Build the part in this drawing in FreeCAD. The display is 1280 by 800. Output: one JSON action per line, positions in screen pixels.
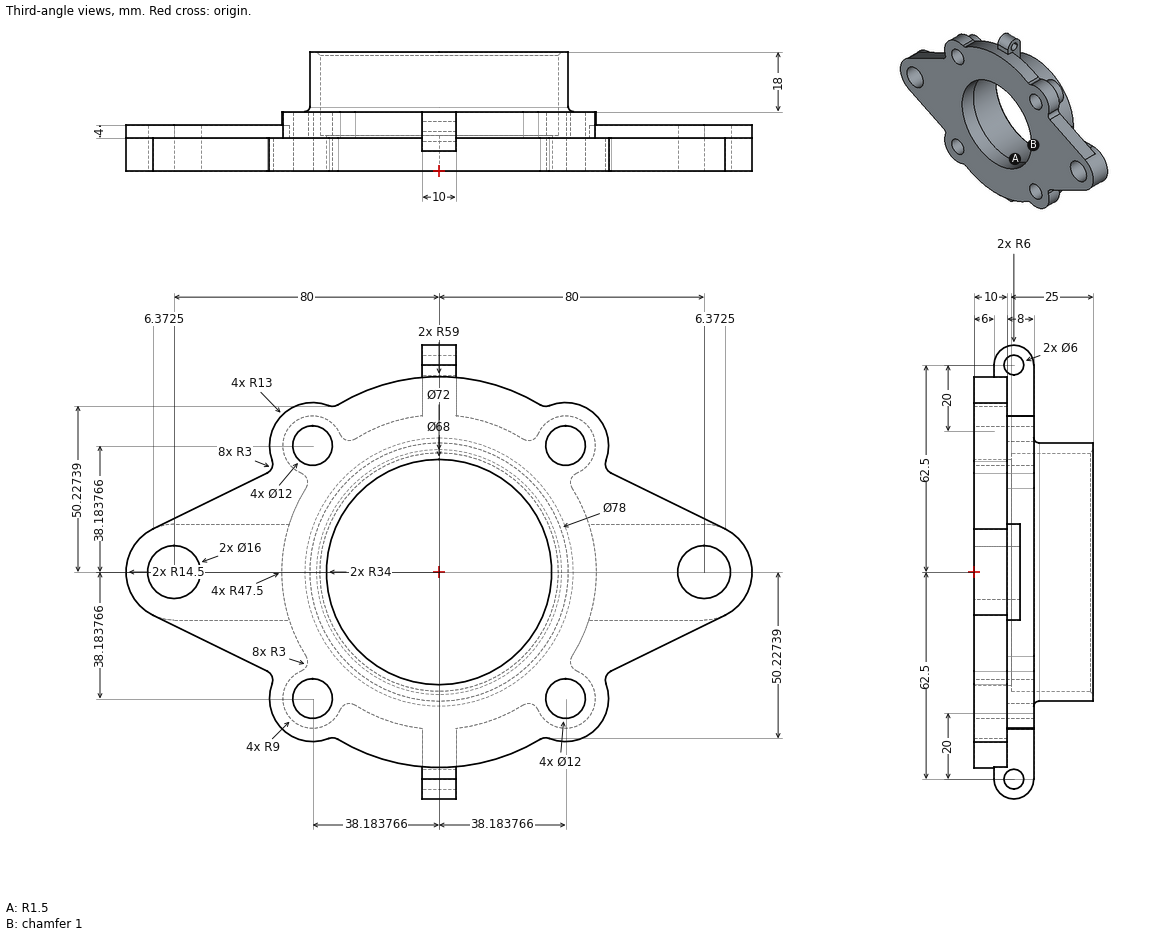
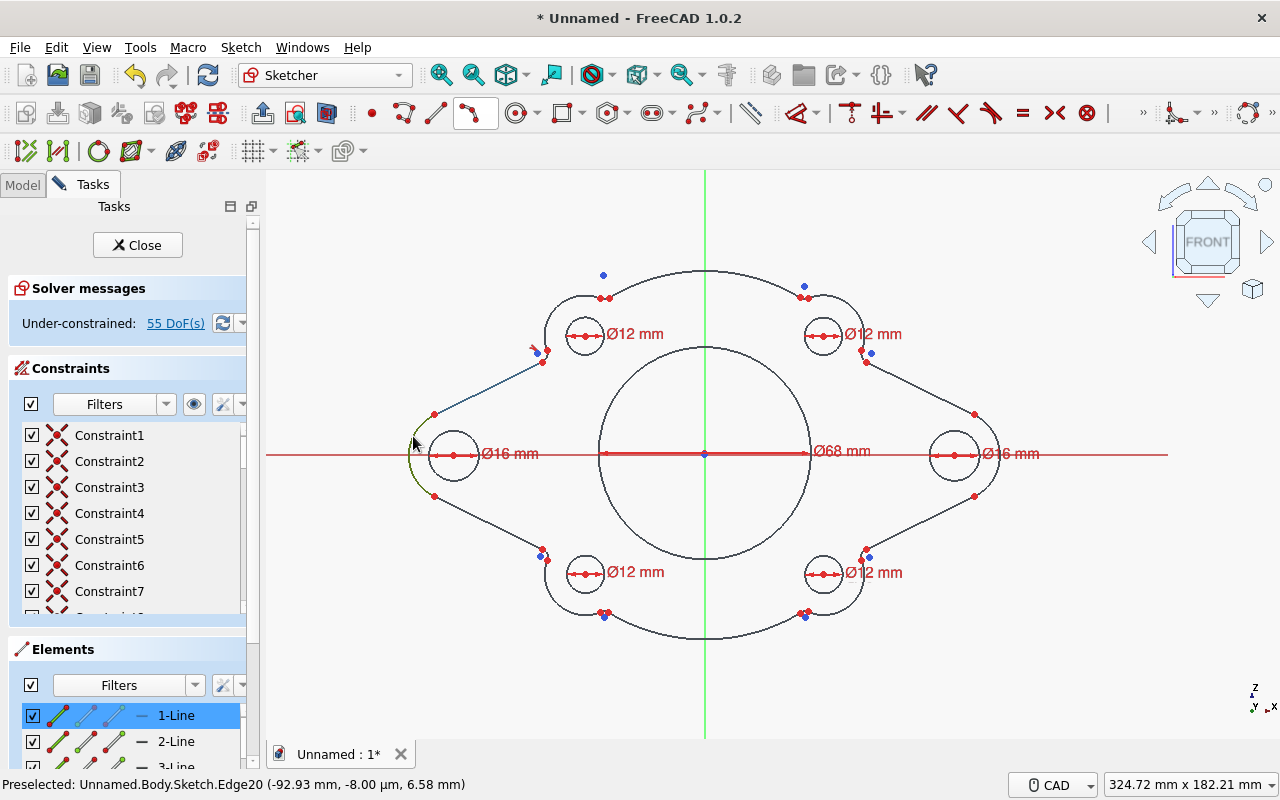
{"action": "left_click", "coordinate": [992, 114]}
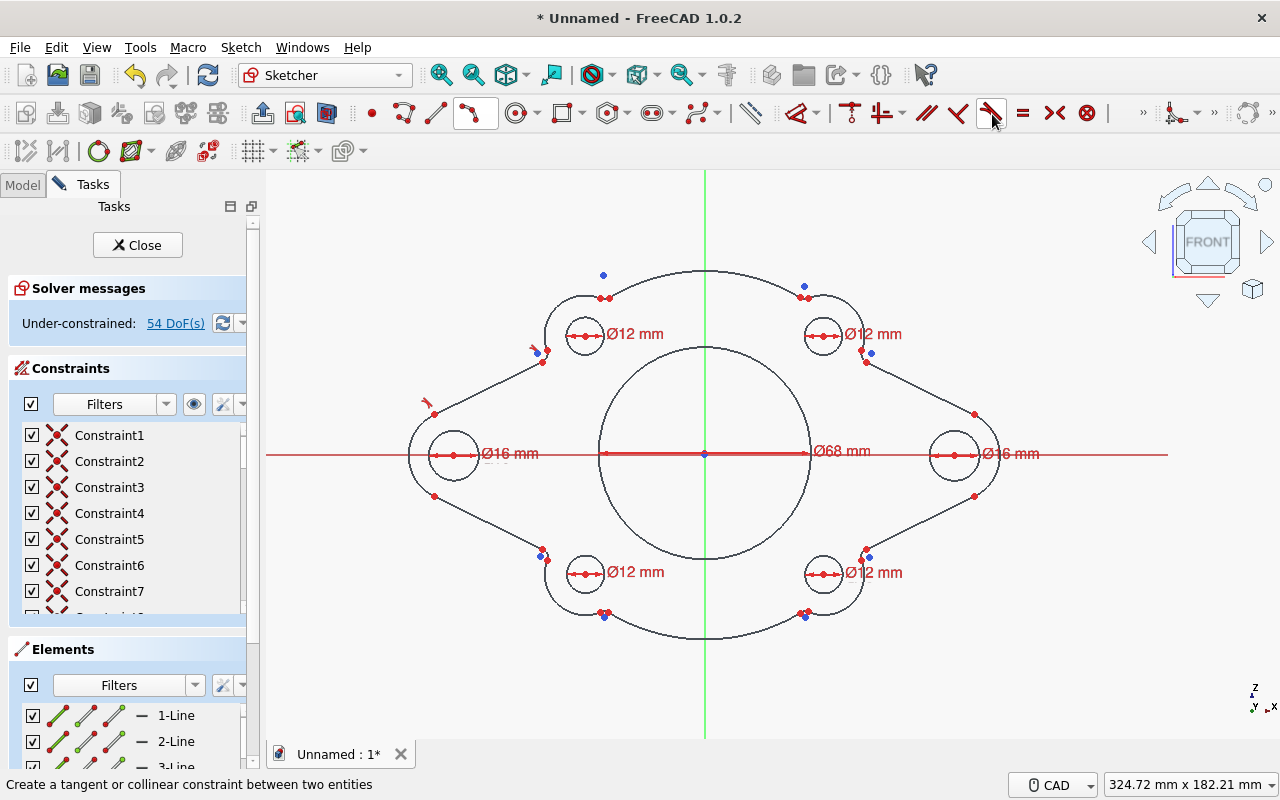
{"action": "left_click", "coordinate": [899, 378]}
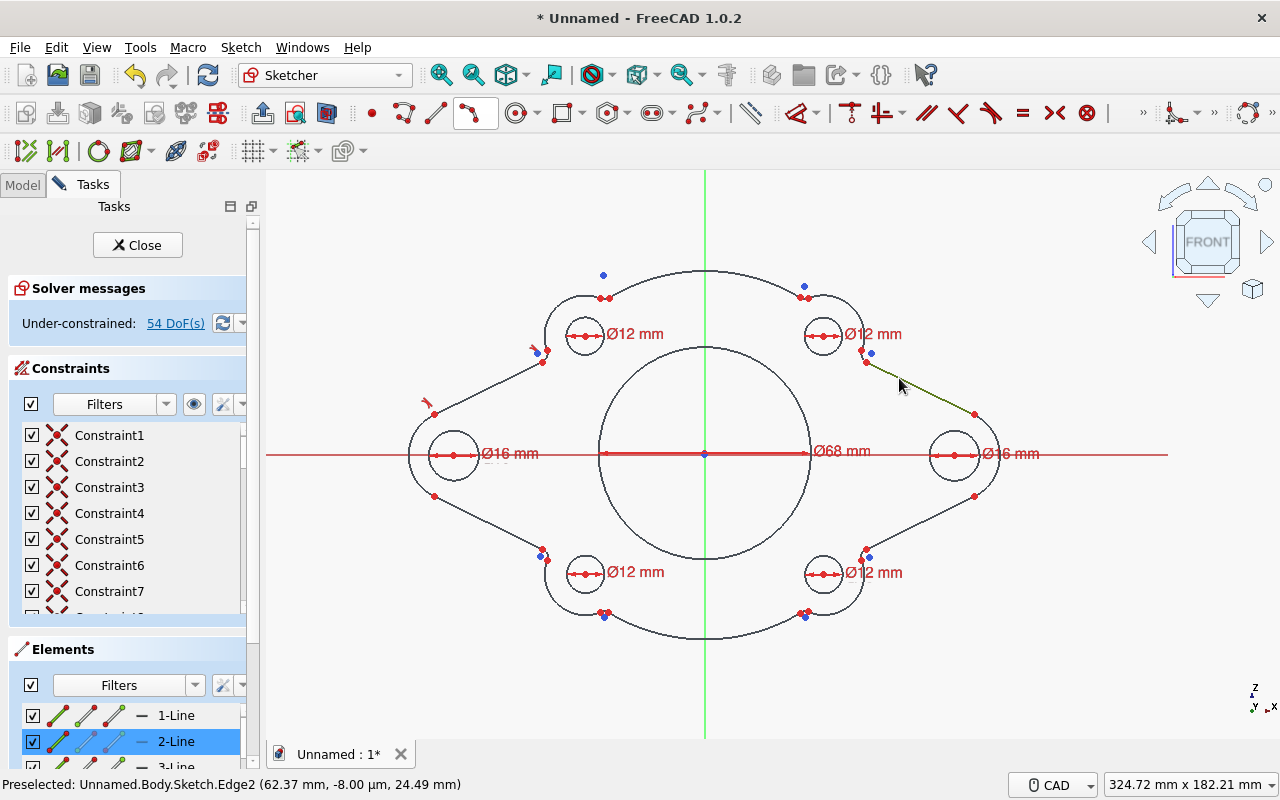
{"action": "scroll", "coordinate": [862, 357], "scroll_direction": "up", "scroll_amount": 4}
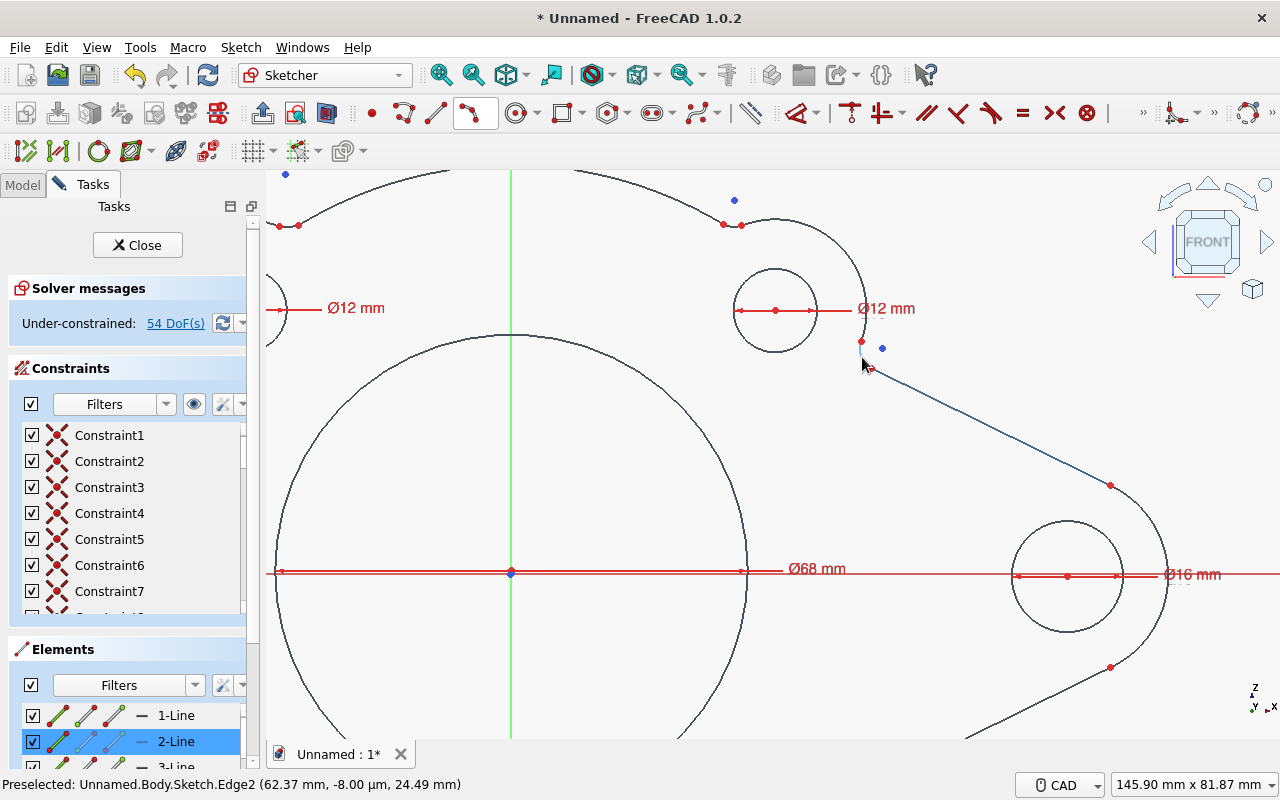
{"action": "left_click", "coordinate": [861, 357]}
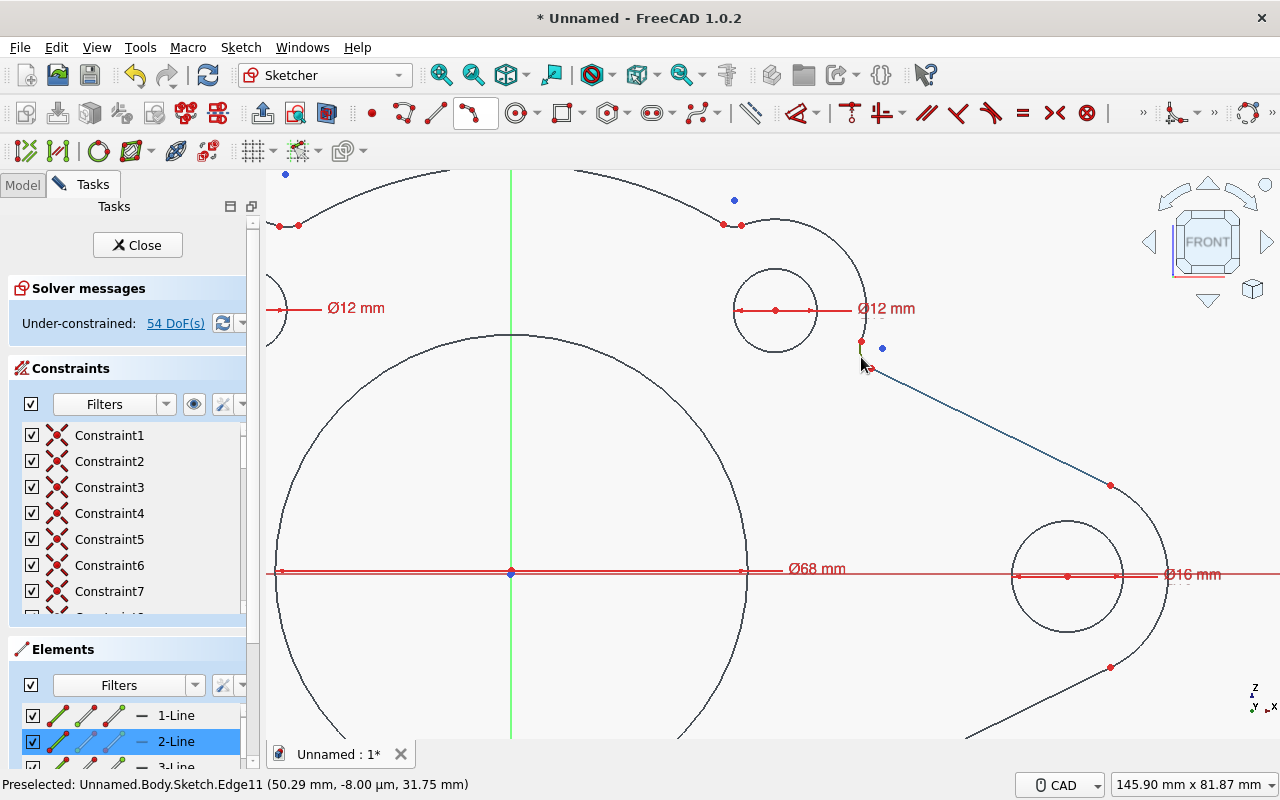
{"action": "left_click", "coordinate": [992, 114]}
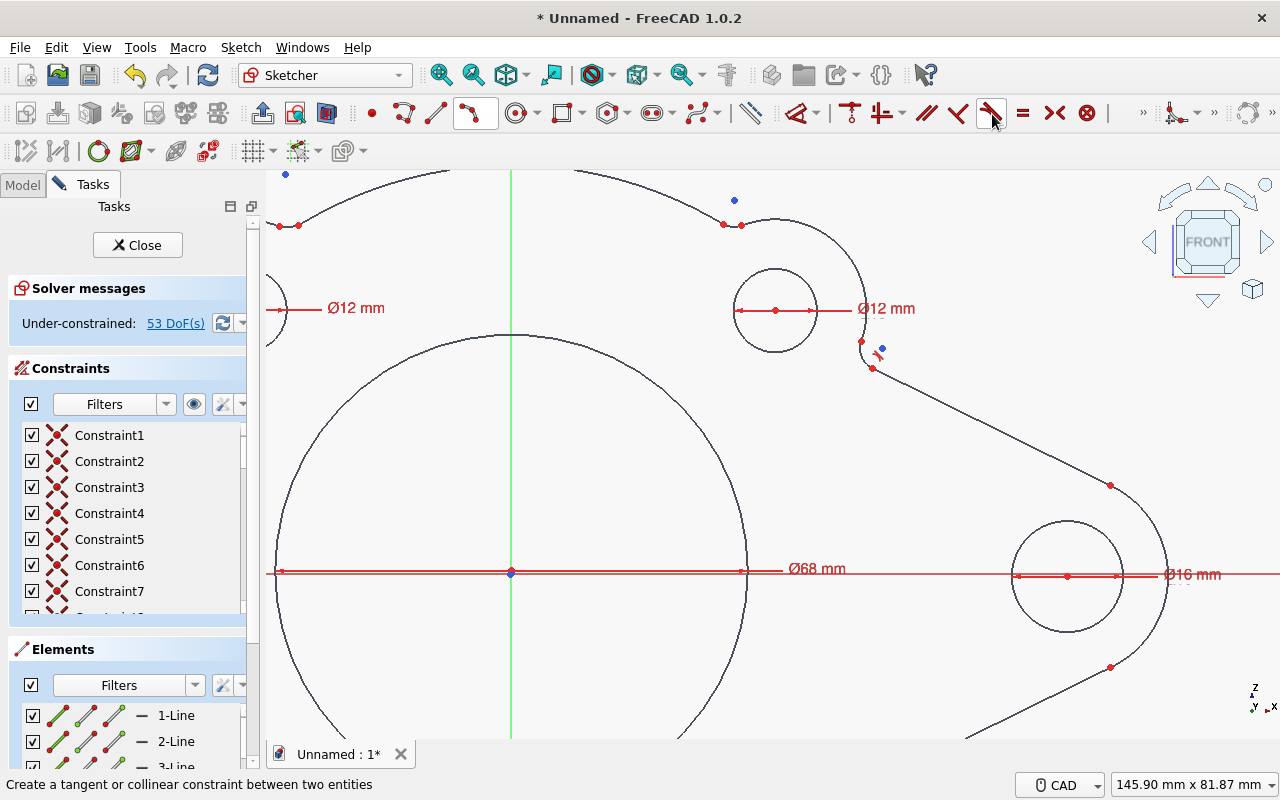
{"action": "left_click", "coordinate": [944, 403]}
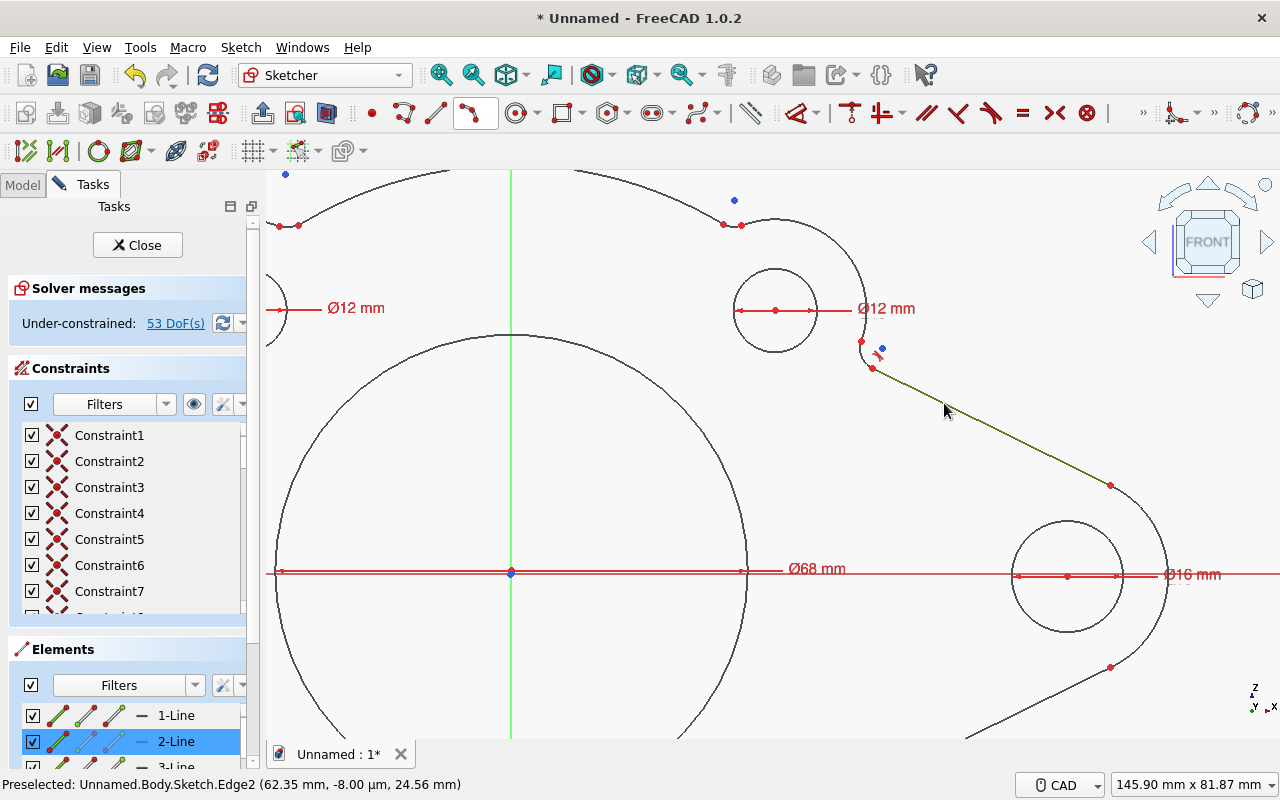
{"action": "scroll", "coordinate": [862, 357], "scroll_direction": "down", "scroll_amount": 4}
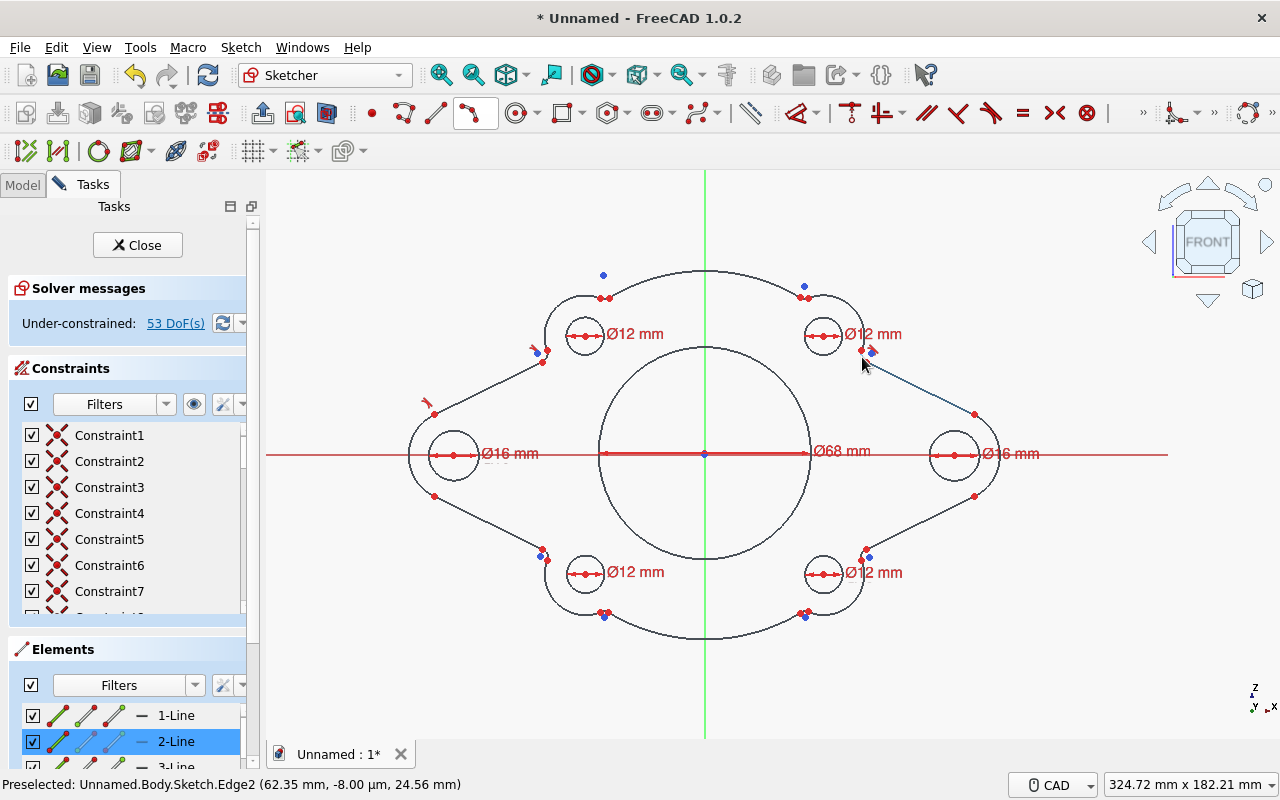
{"action": "left_click", "coordinate": [995, 476]}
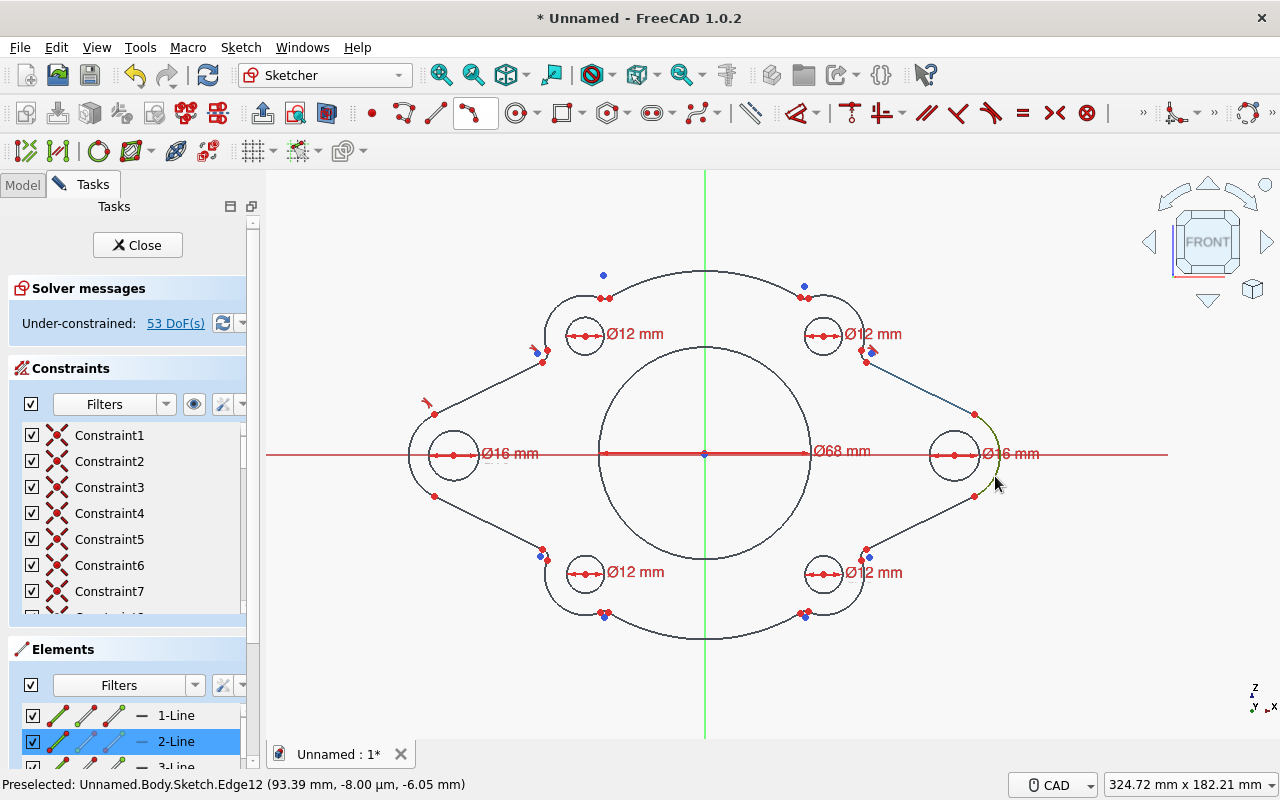
{"action": "left_click", "coordinate": [992, 114]}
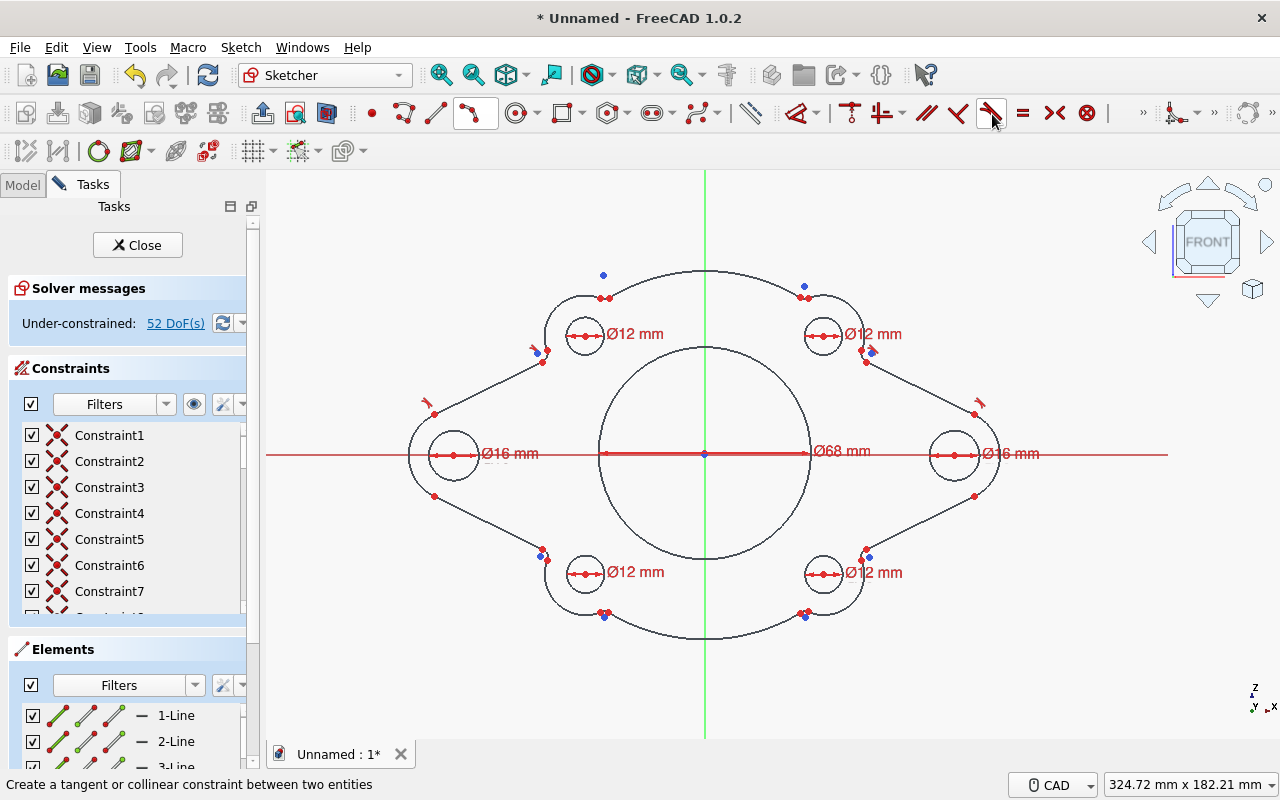
{"action": "left_click", "coordinate": [942, 513]}